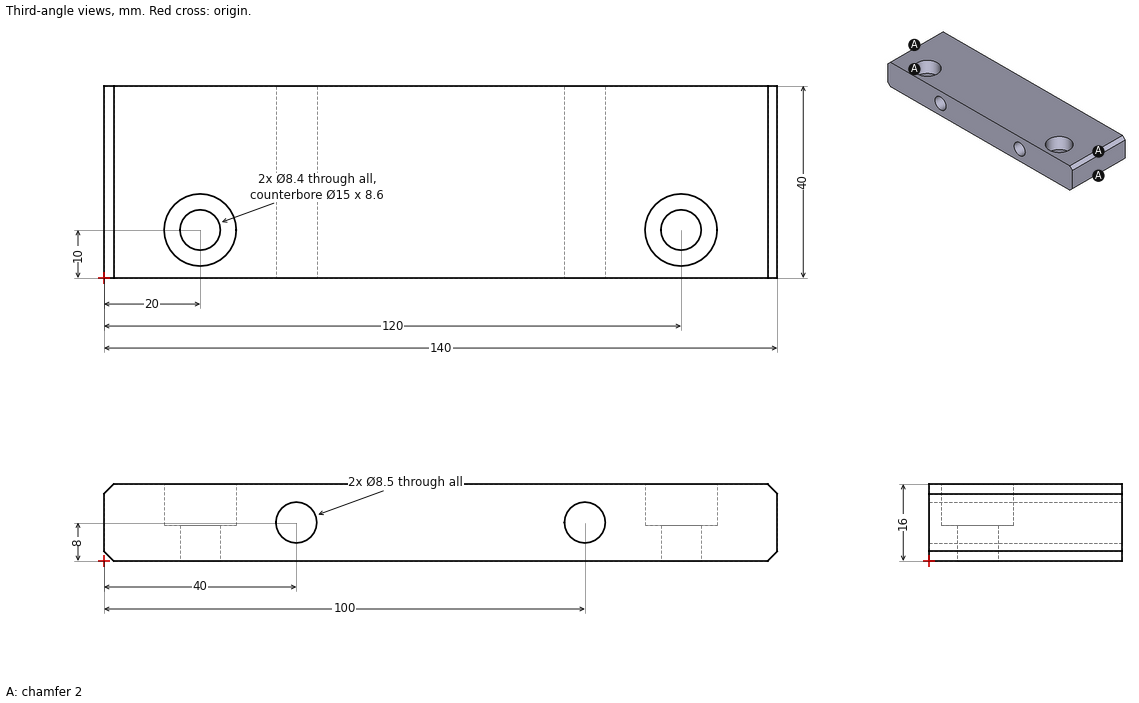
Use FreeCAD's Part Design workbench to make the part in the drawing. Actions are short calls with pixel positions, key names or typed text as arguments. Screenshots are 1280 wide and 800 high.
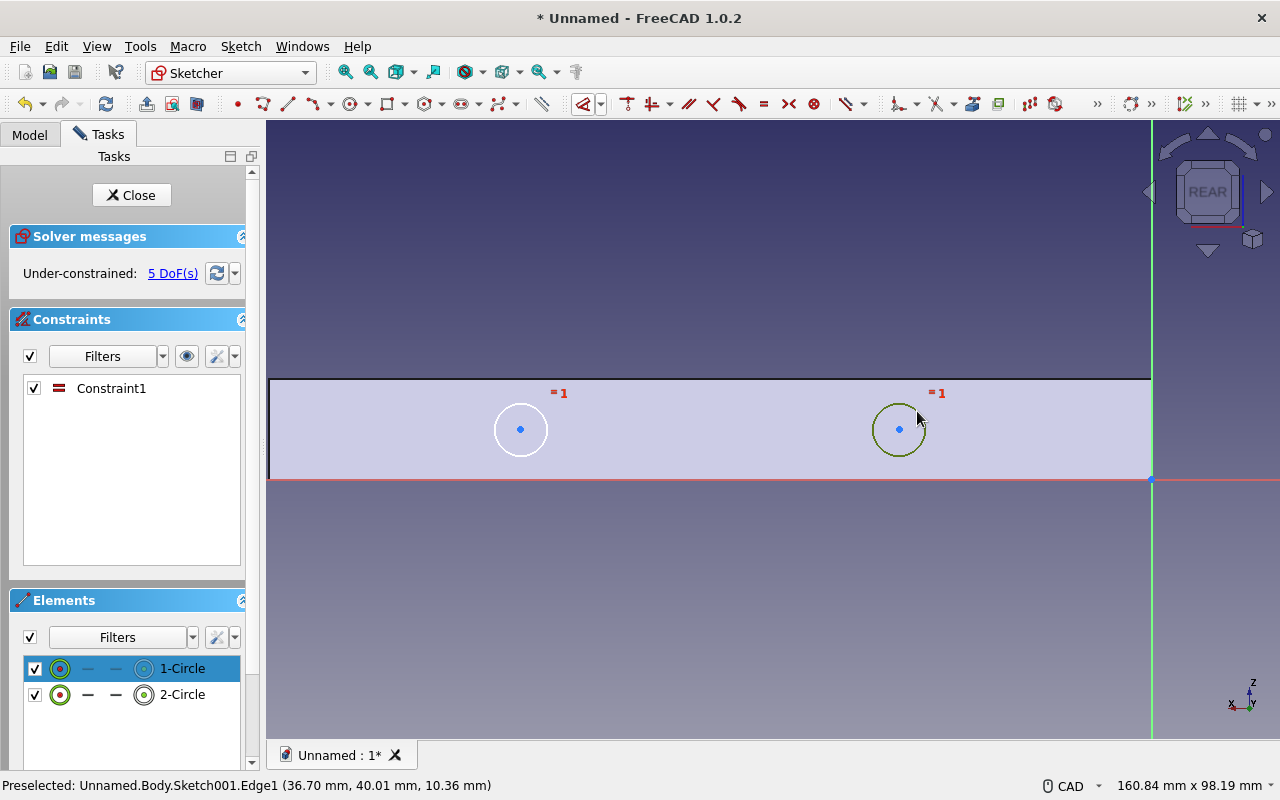
click(600, 104)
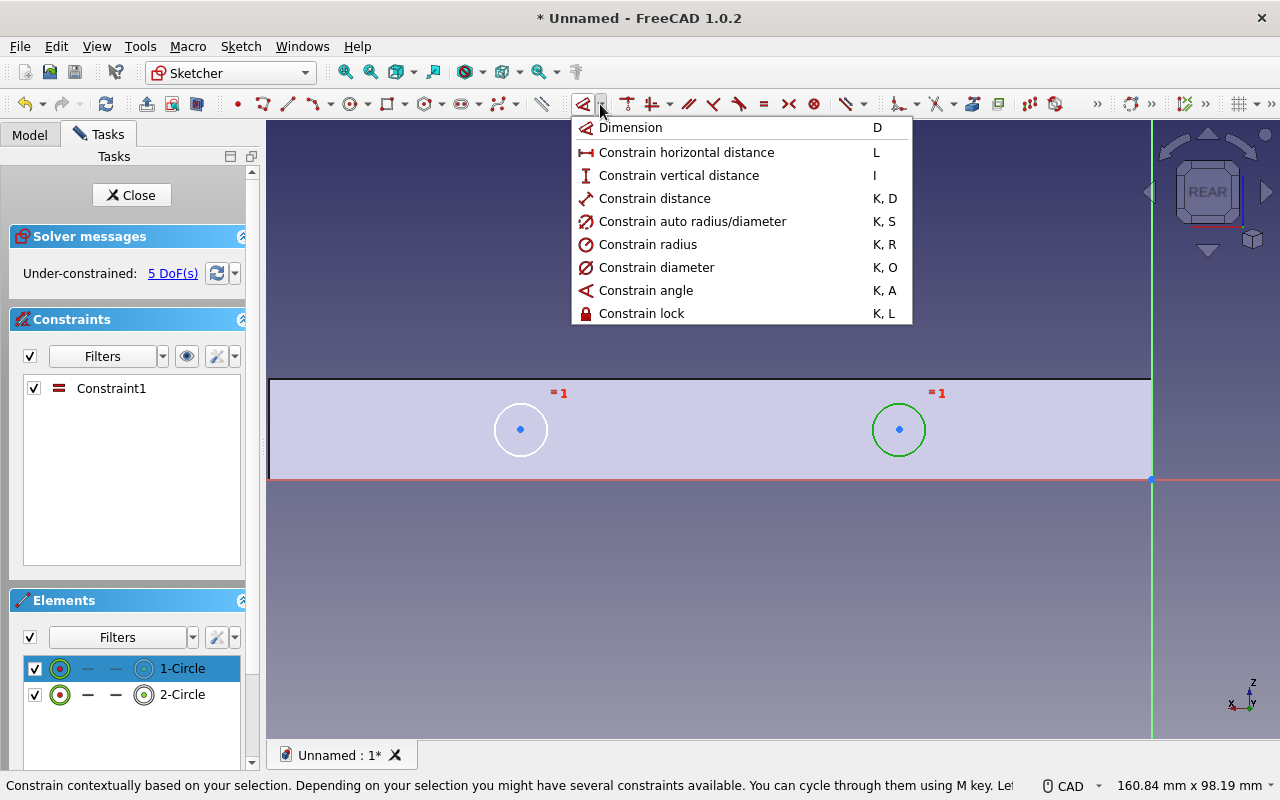
click(742, 268)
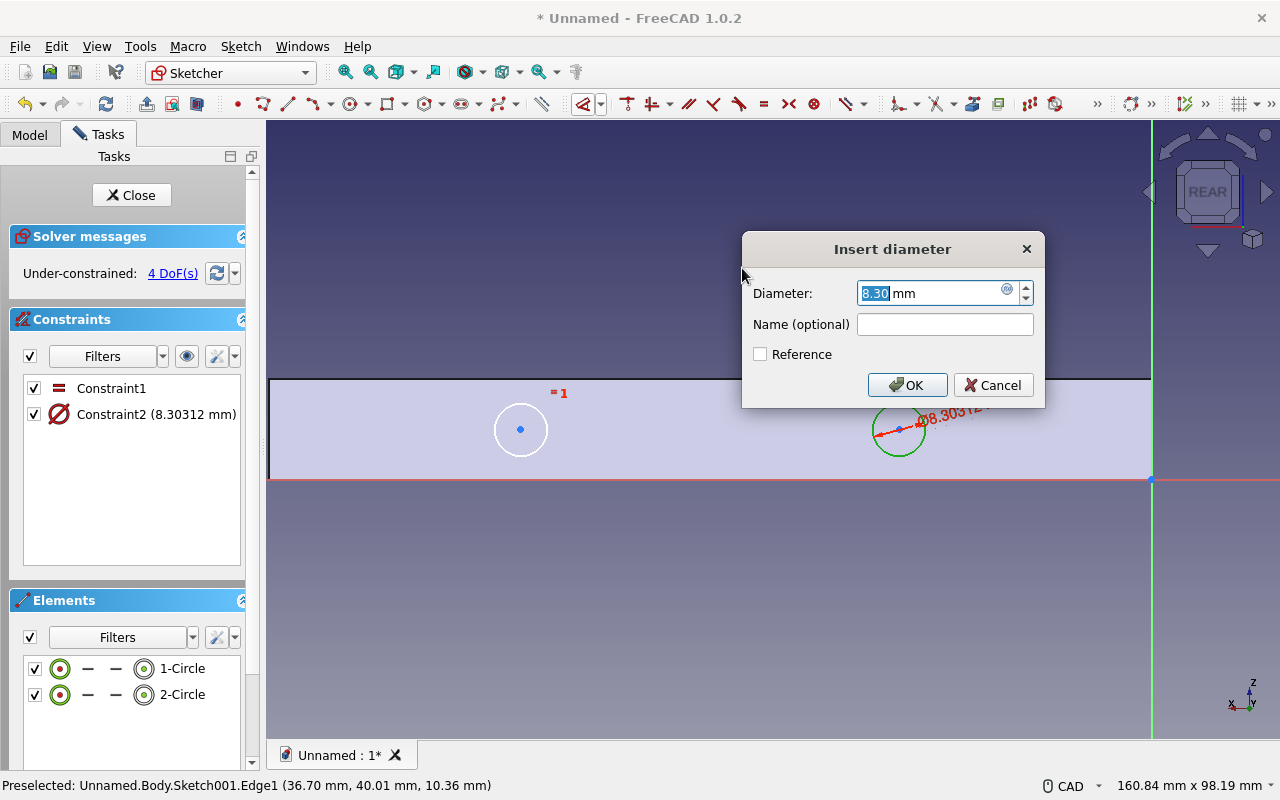
text(8.5)
key(Return)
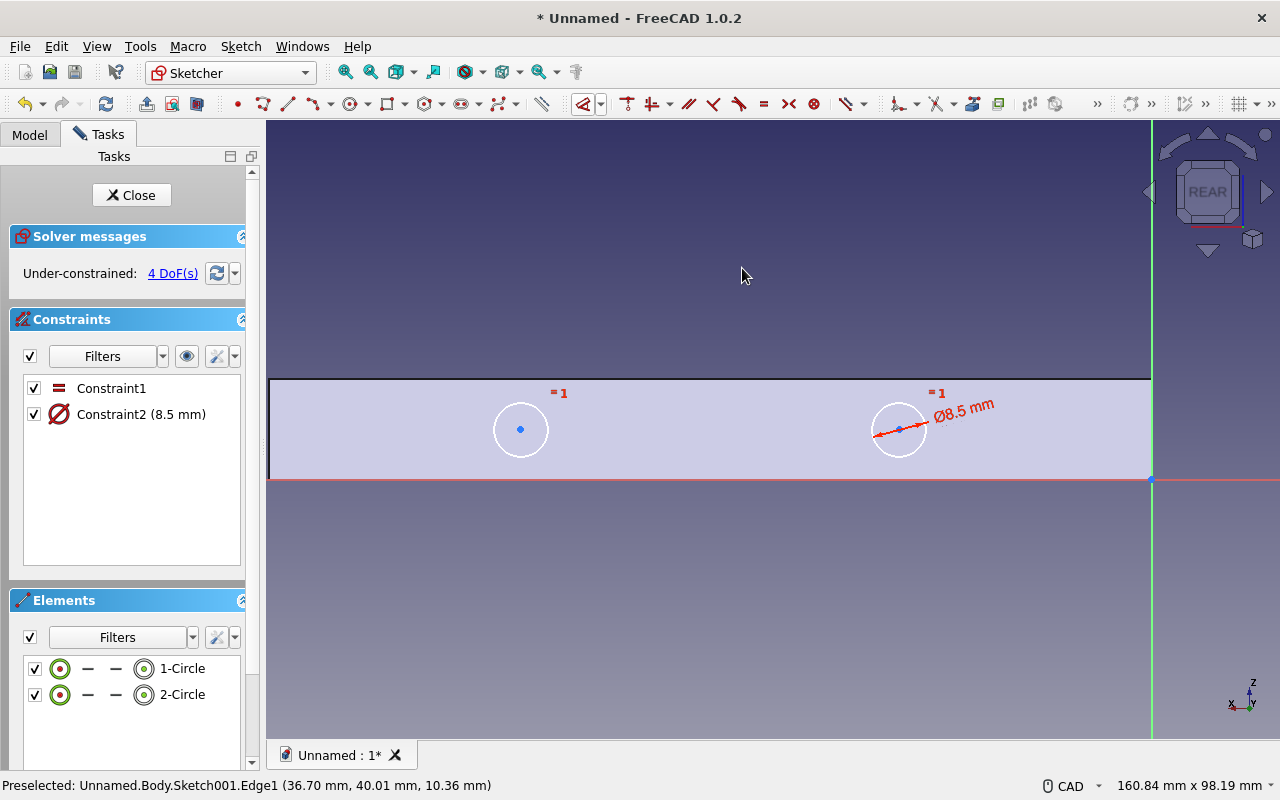
click(899, 430)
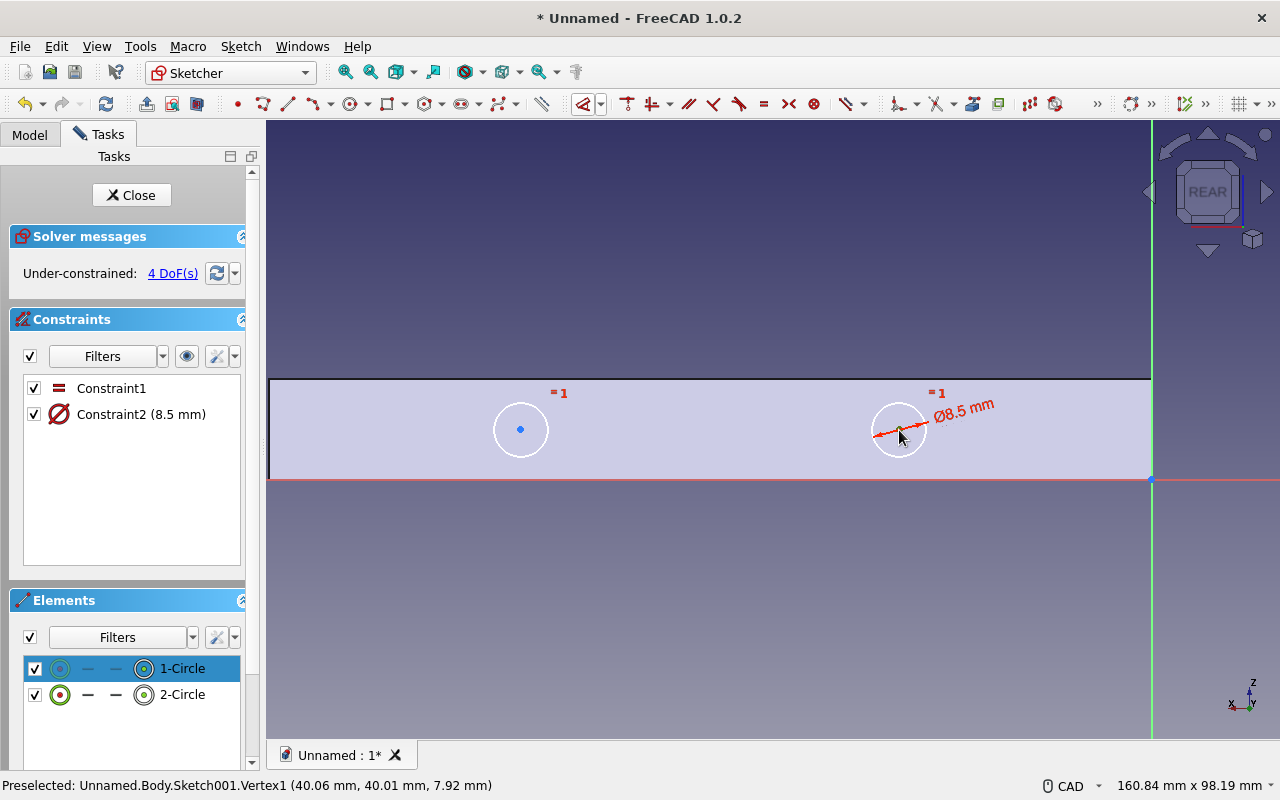
click(600, 104)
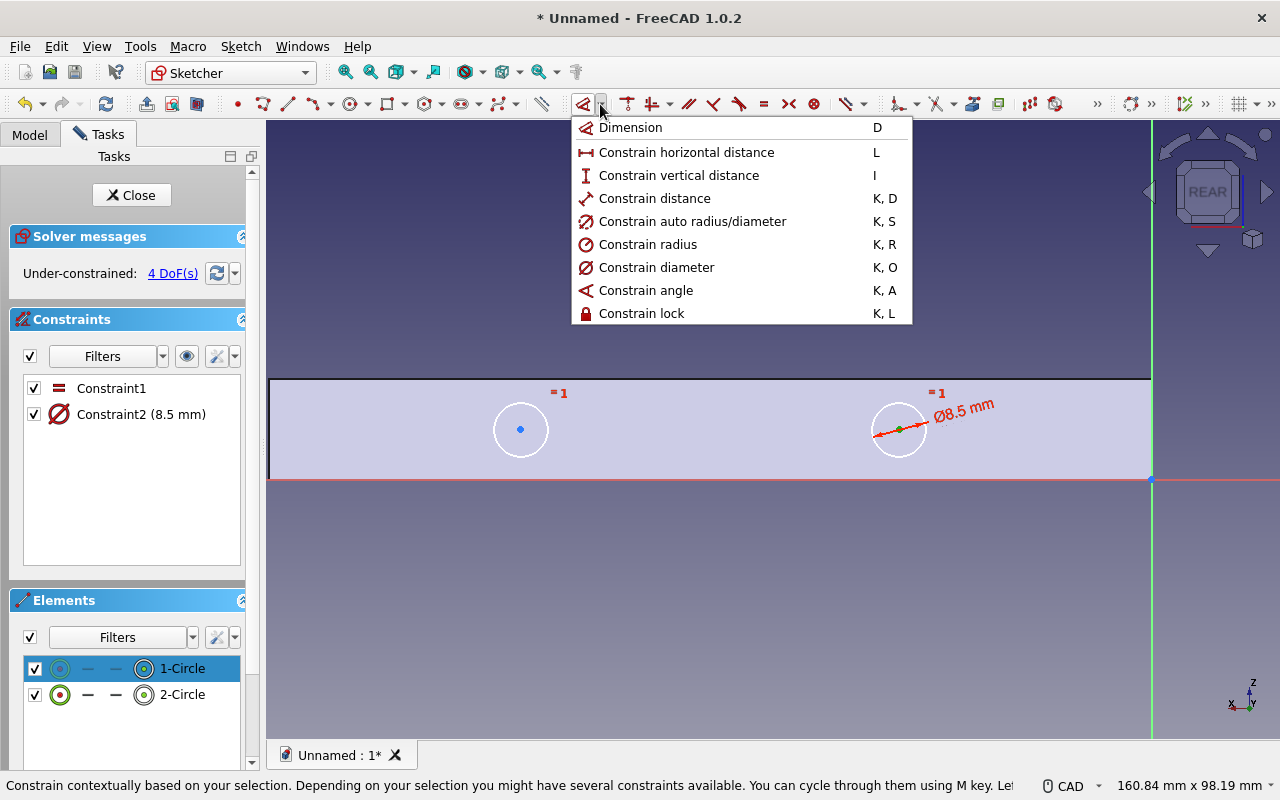
click(742, 176)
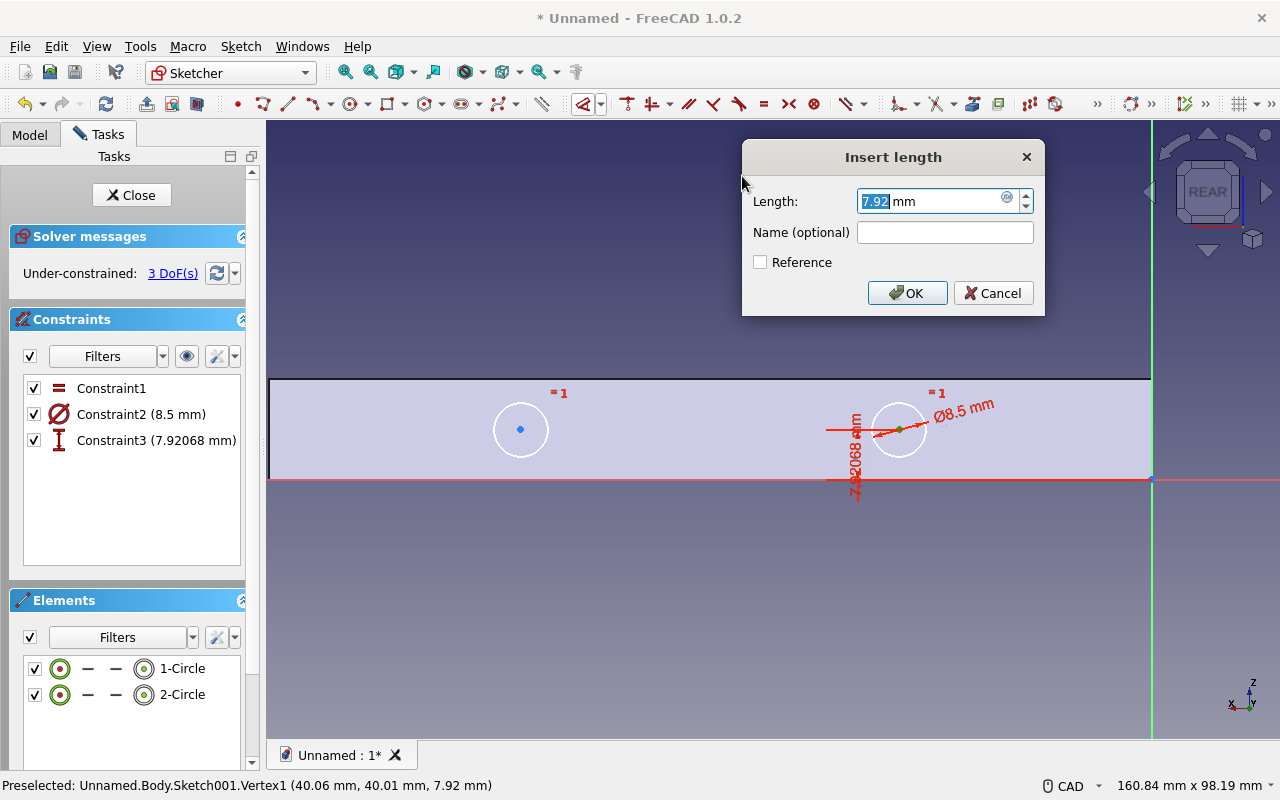
text(8)
key(Return)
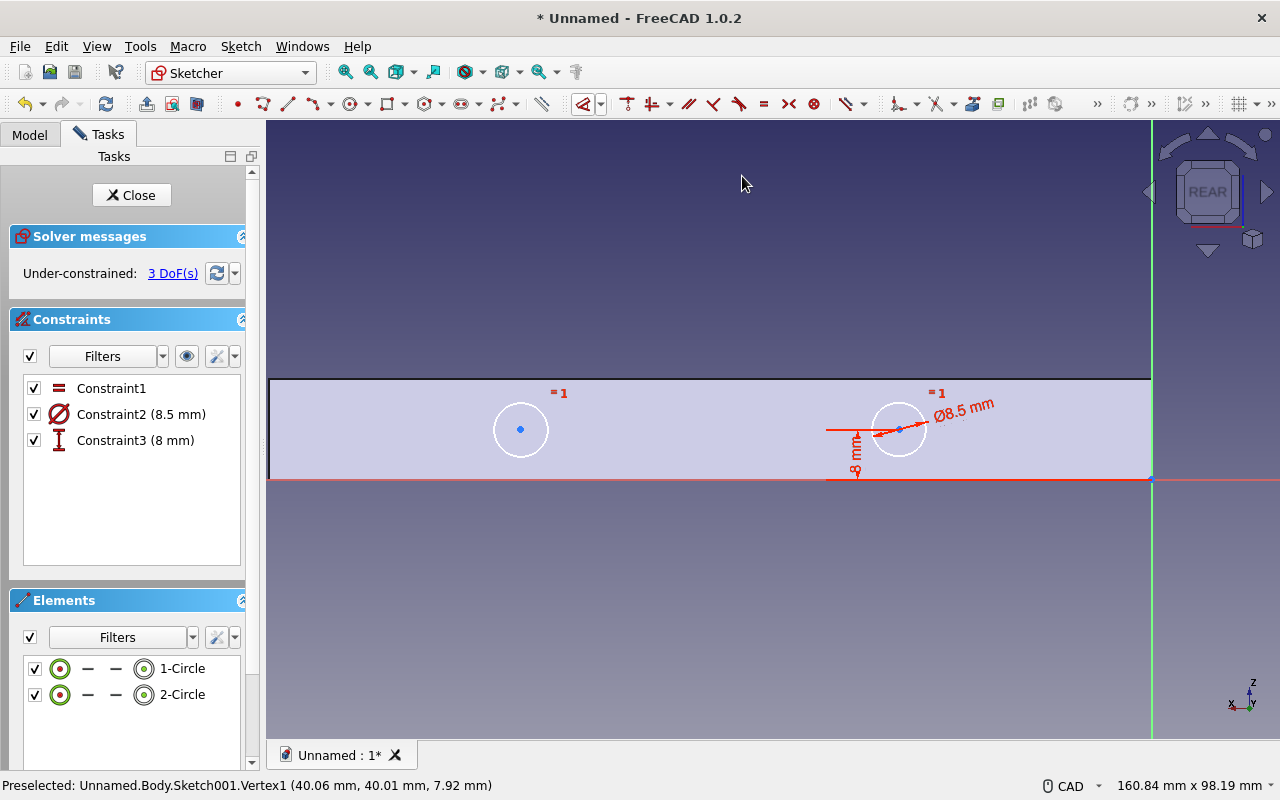
click(521, 430)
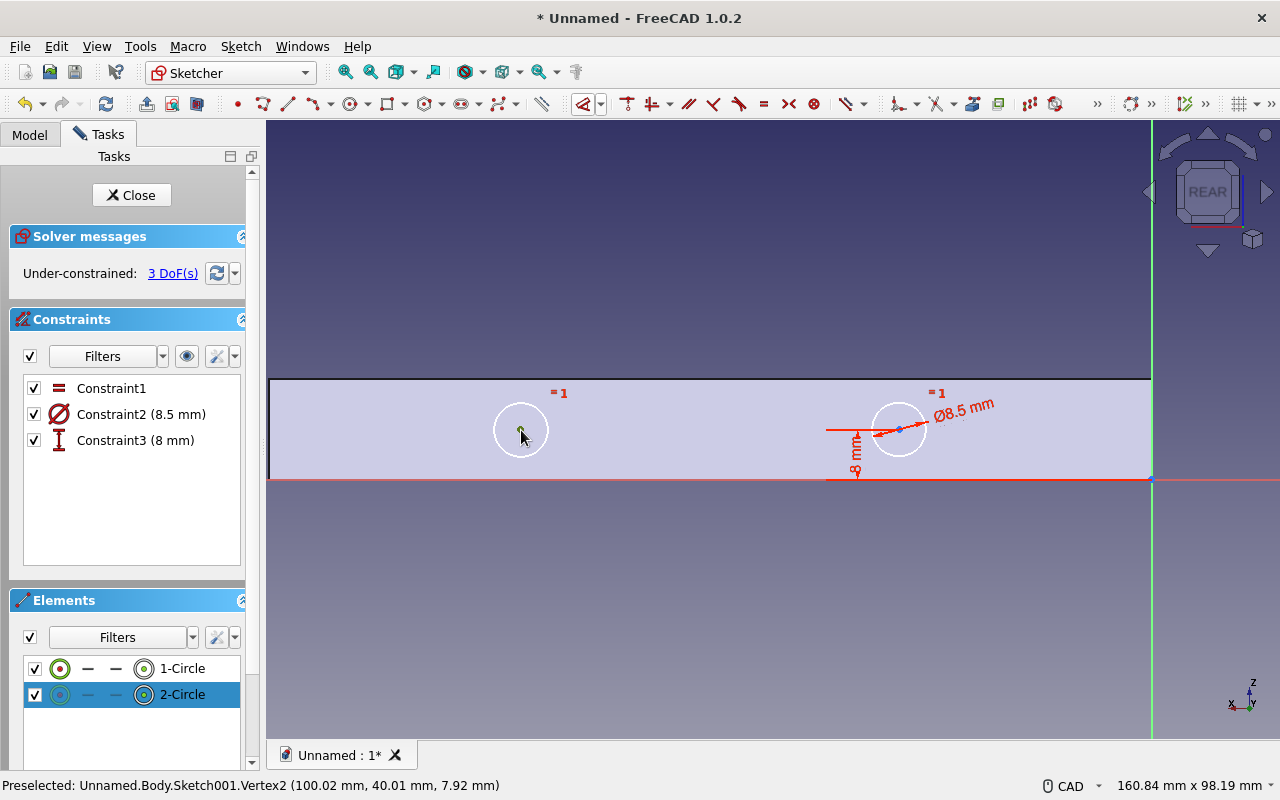
key(i)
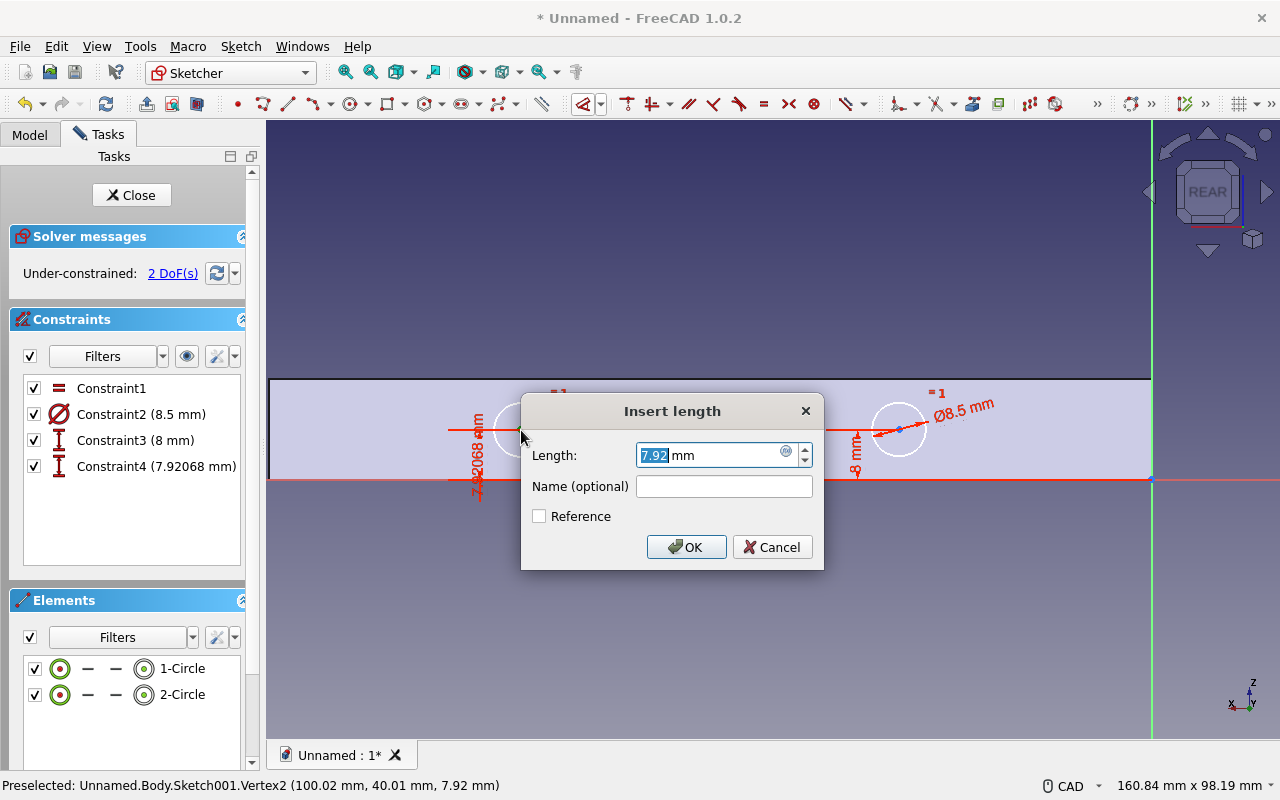
text(8)
key(Return)